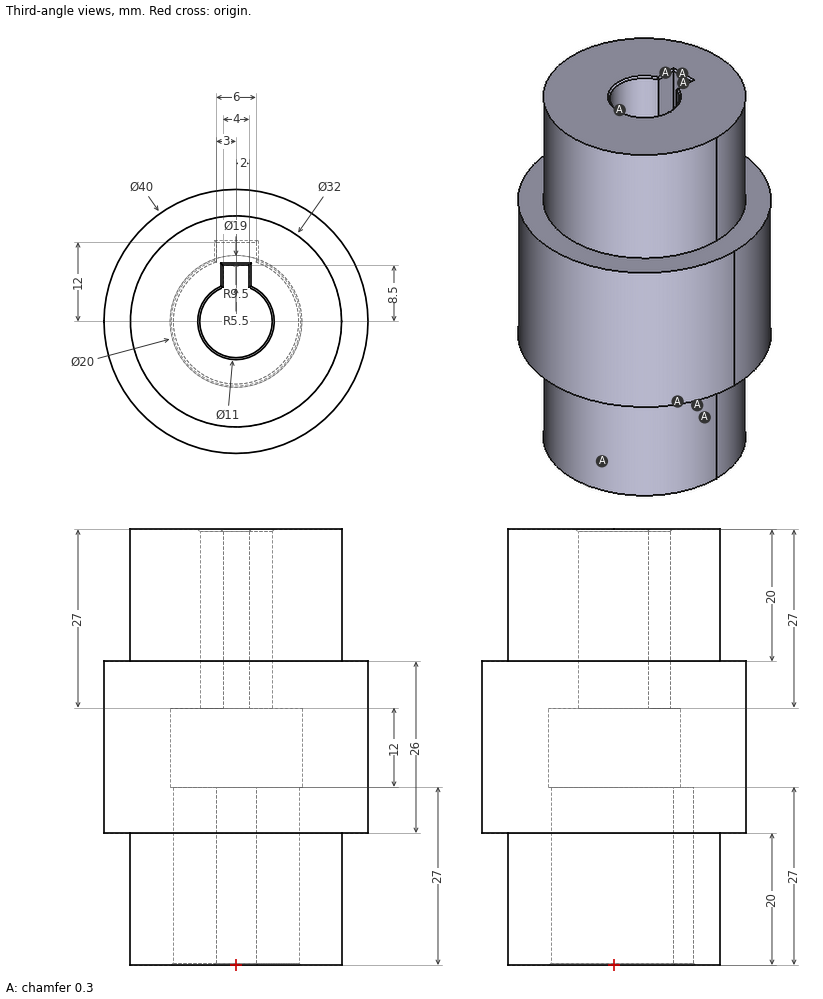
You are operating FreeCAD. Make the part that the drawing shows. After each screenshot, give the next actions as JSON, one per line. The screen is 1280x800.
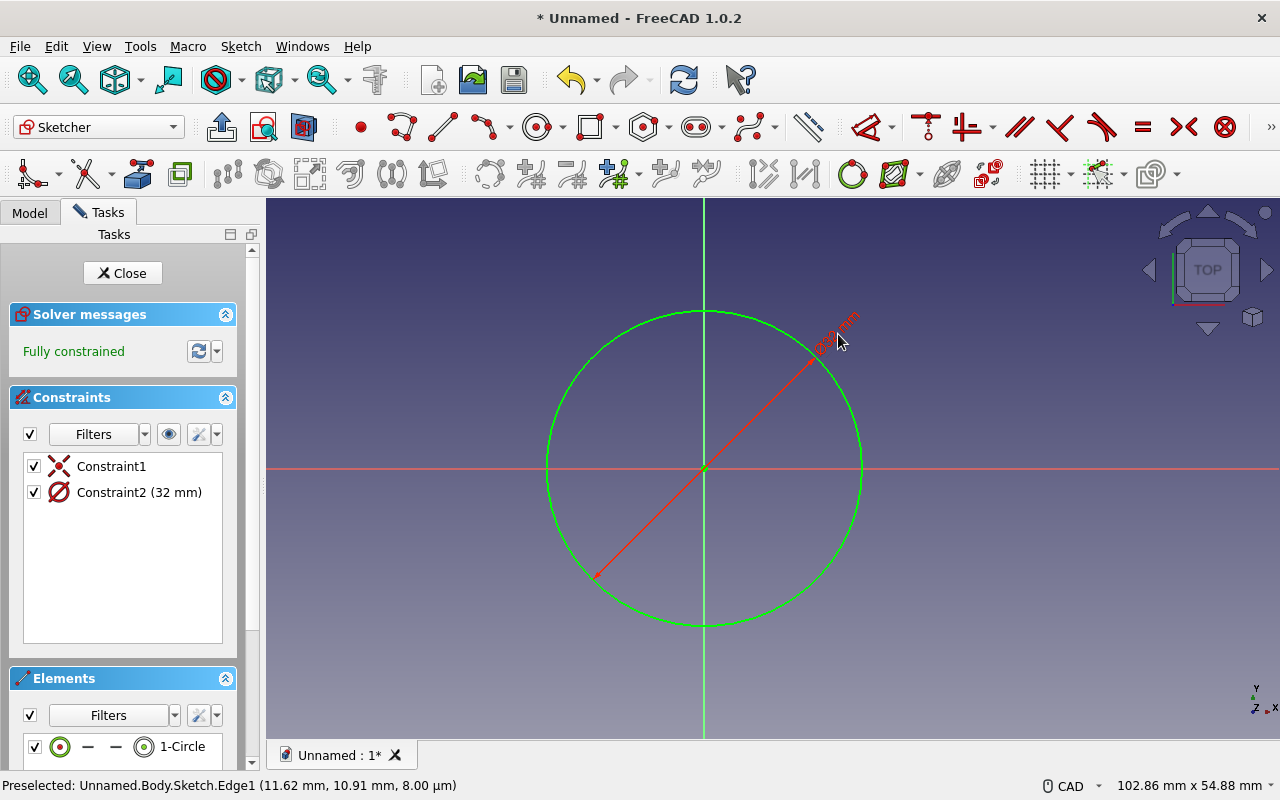
{"action": "left_click", "coordinate": [123, 273]}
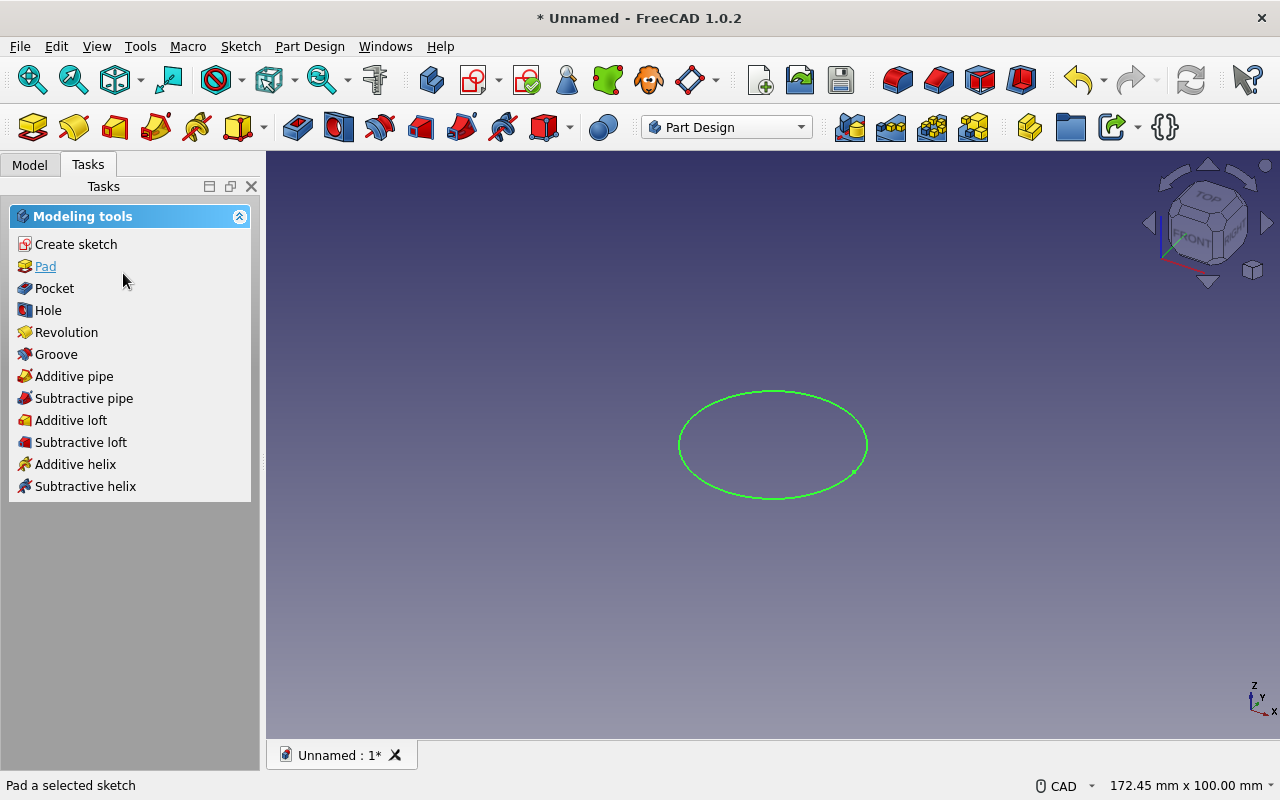
{"action": "left_click", "coordinate": [33, 128]}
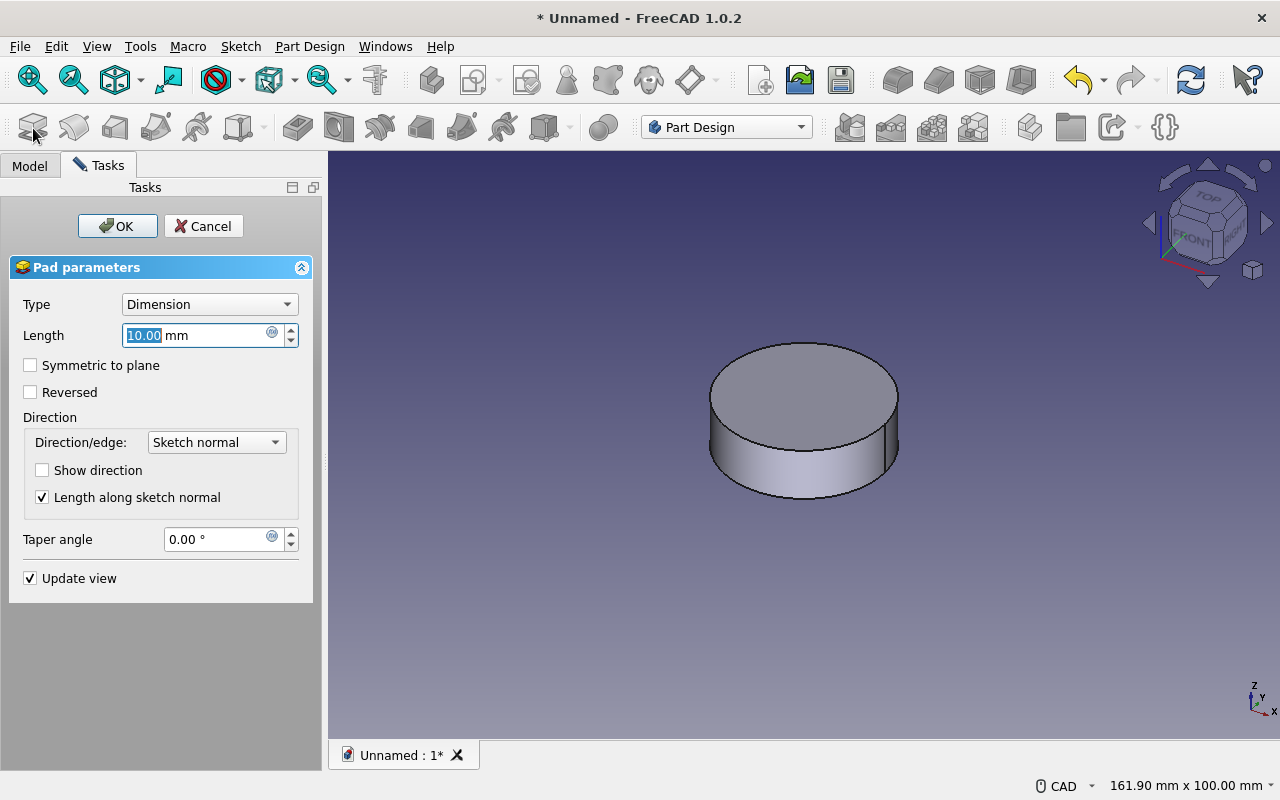
{"action": "type", "text": "20"}
{"action": "key", "text": "Tab"}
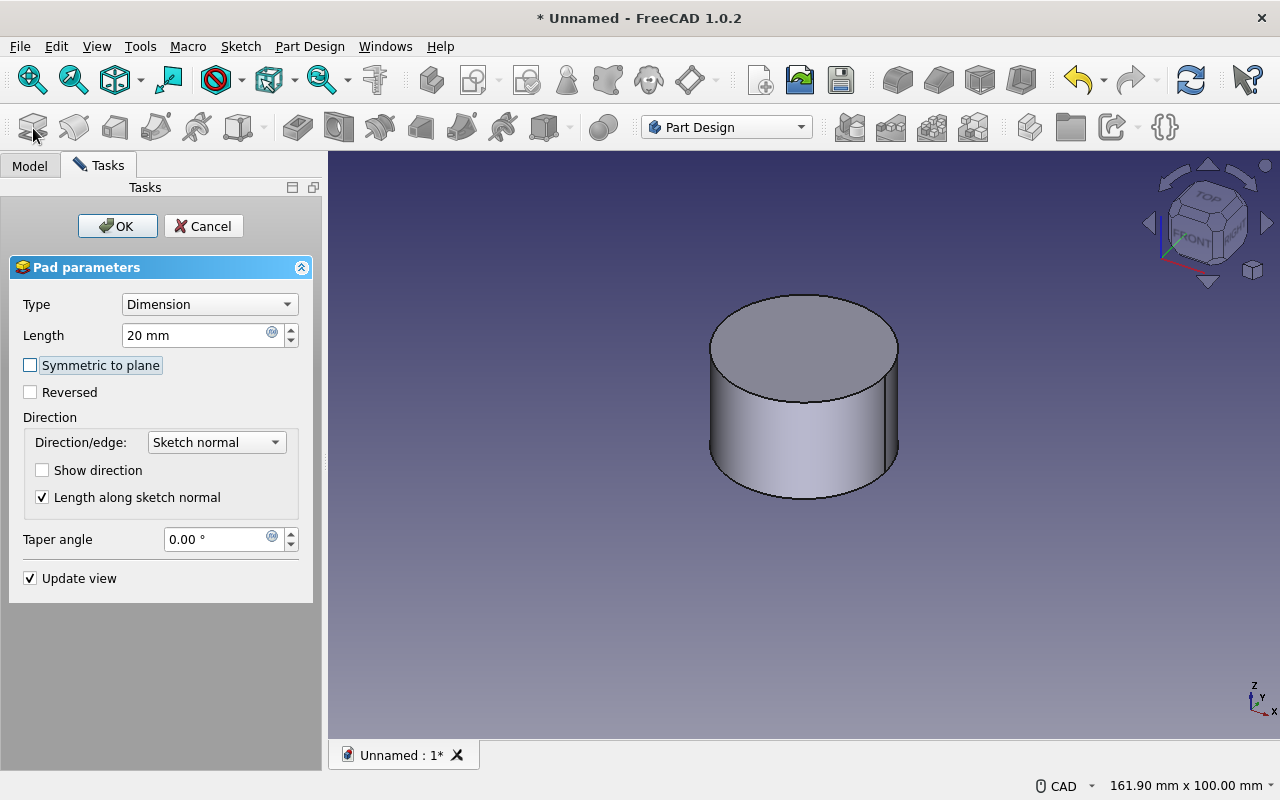
{"action": "left_click", "coordinate": [118, 226]}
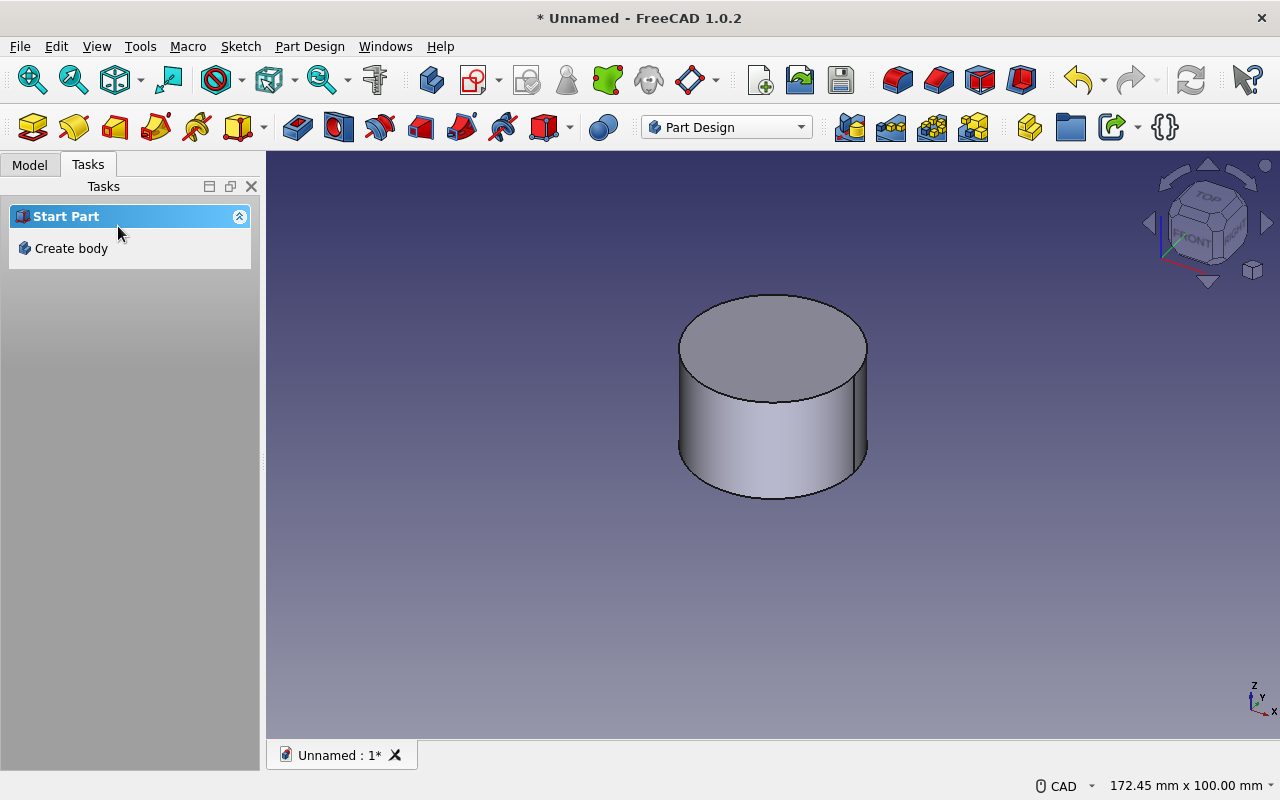
{"action": "left_click", "coordinate": [33, 80]}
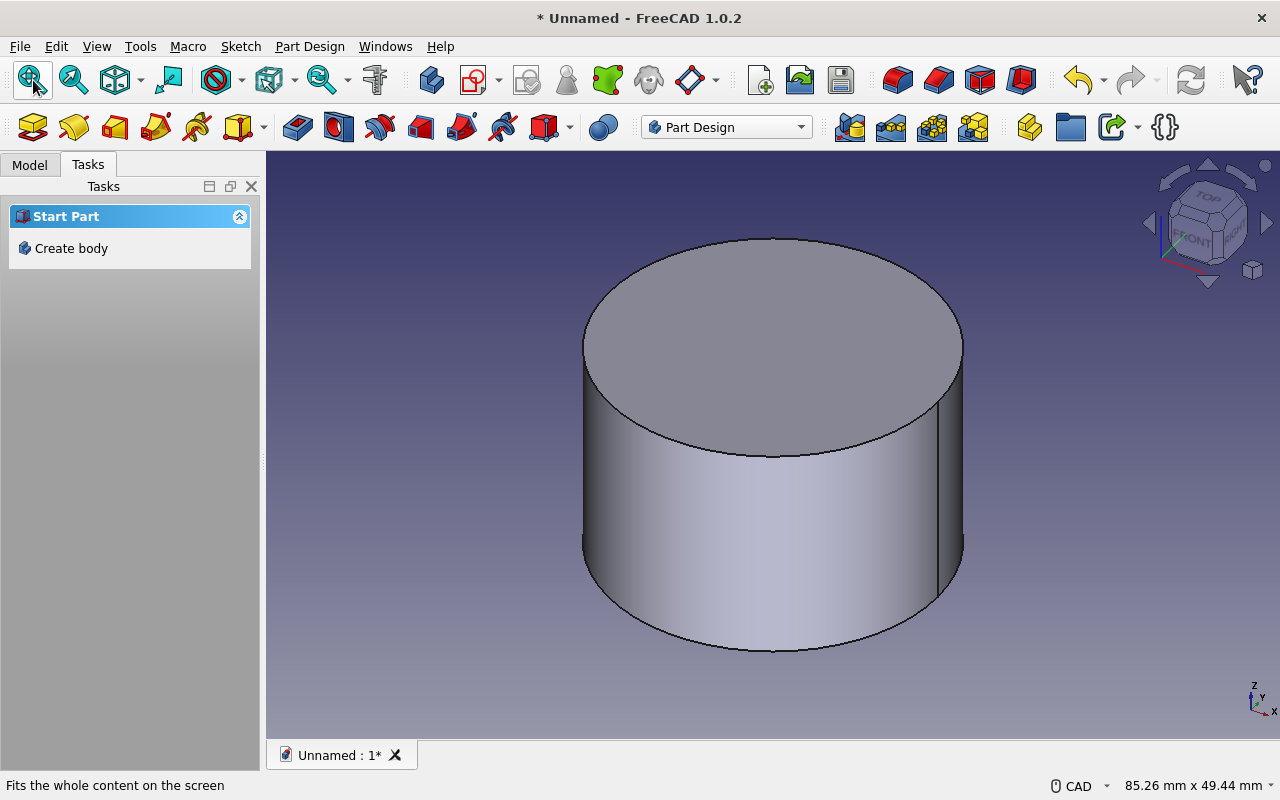
{"action": "left_click", "coordinate": [773, 347]}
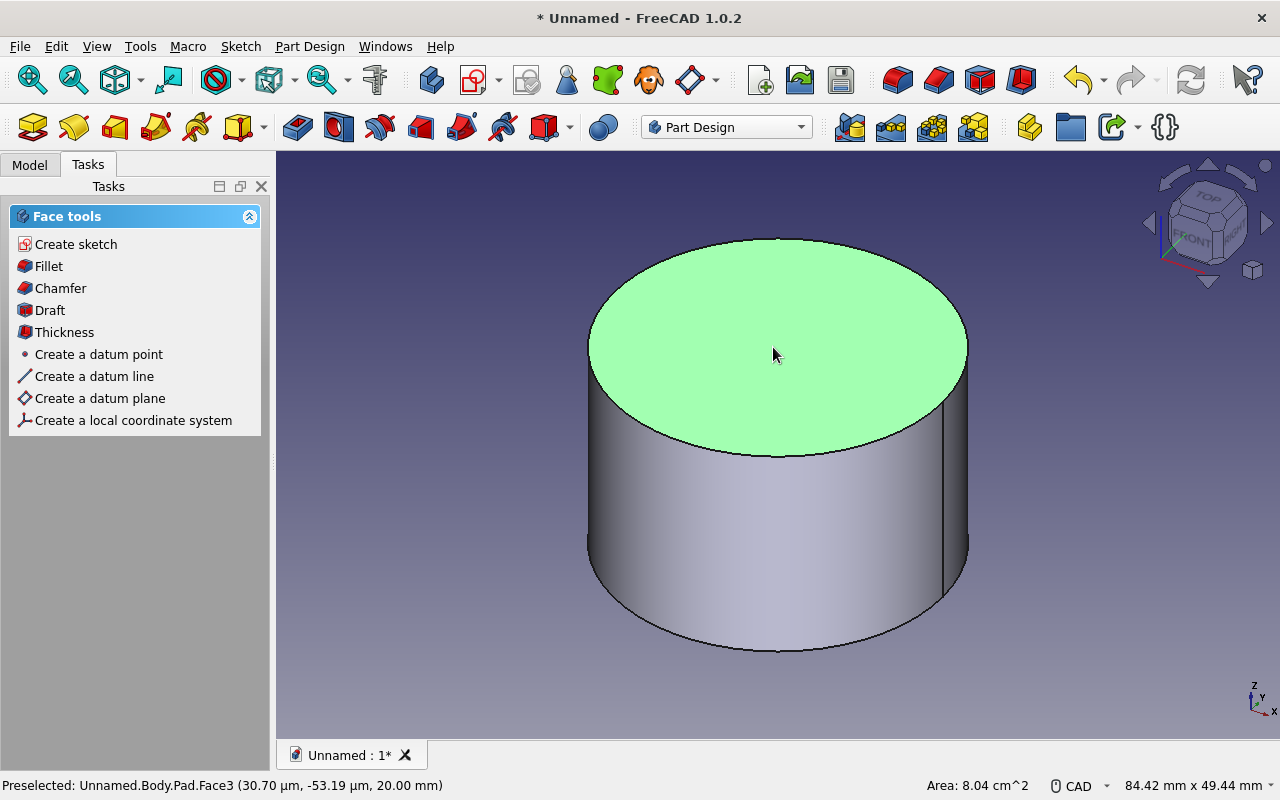
{"action": "left_click", "coordinate": [472, 80]}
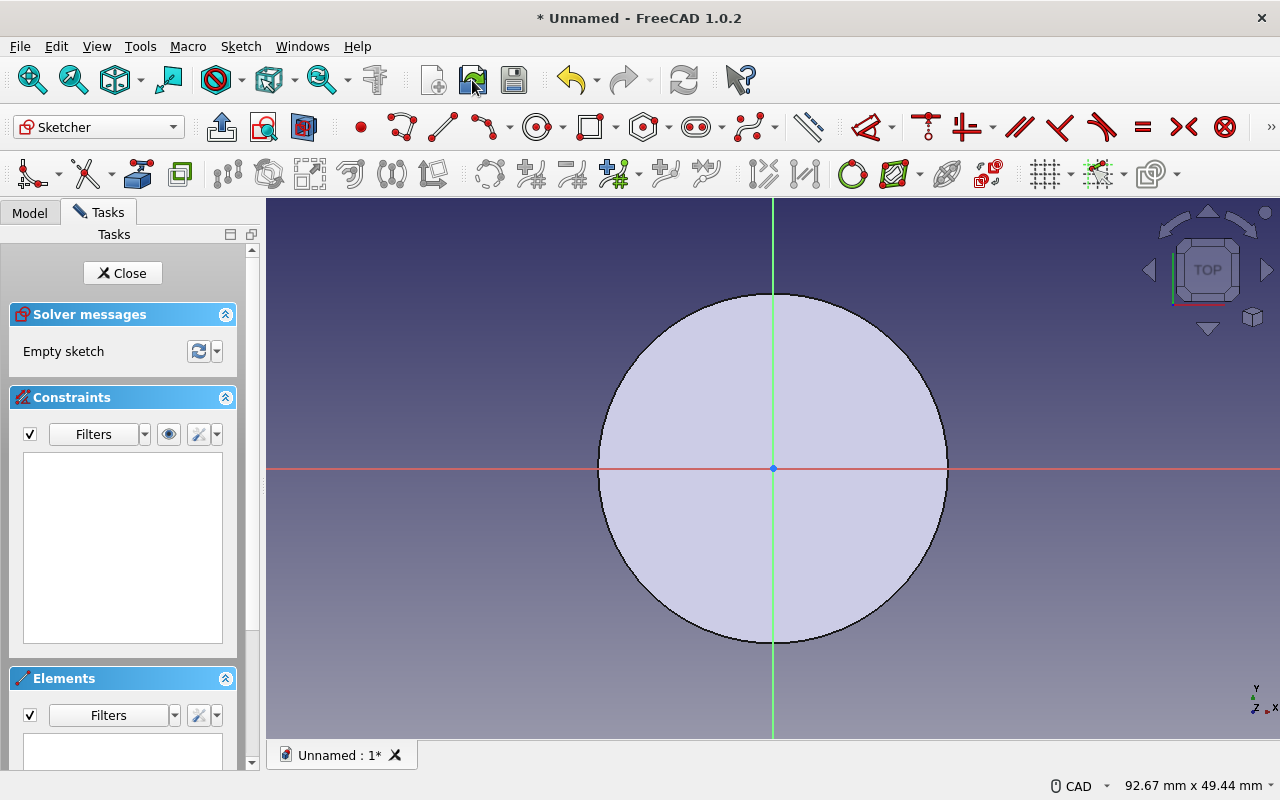
{"action": "scroll", "coordinate": [395, 468], "scroll_direction": "down", "scroll_amount": 1}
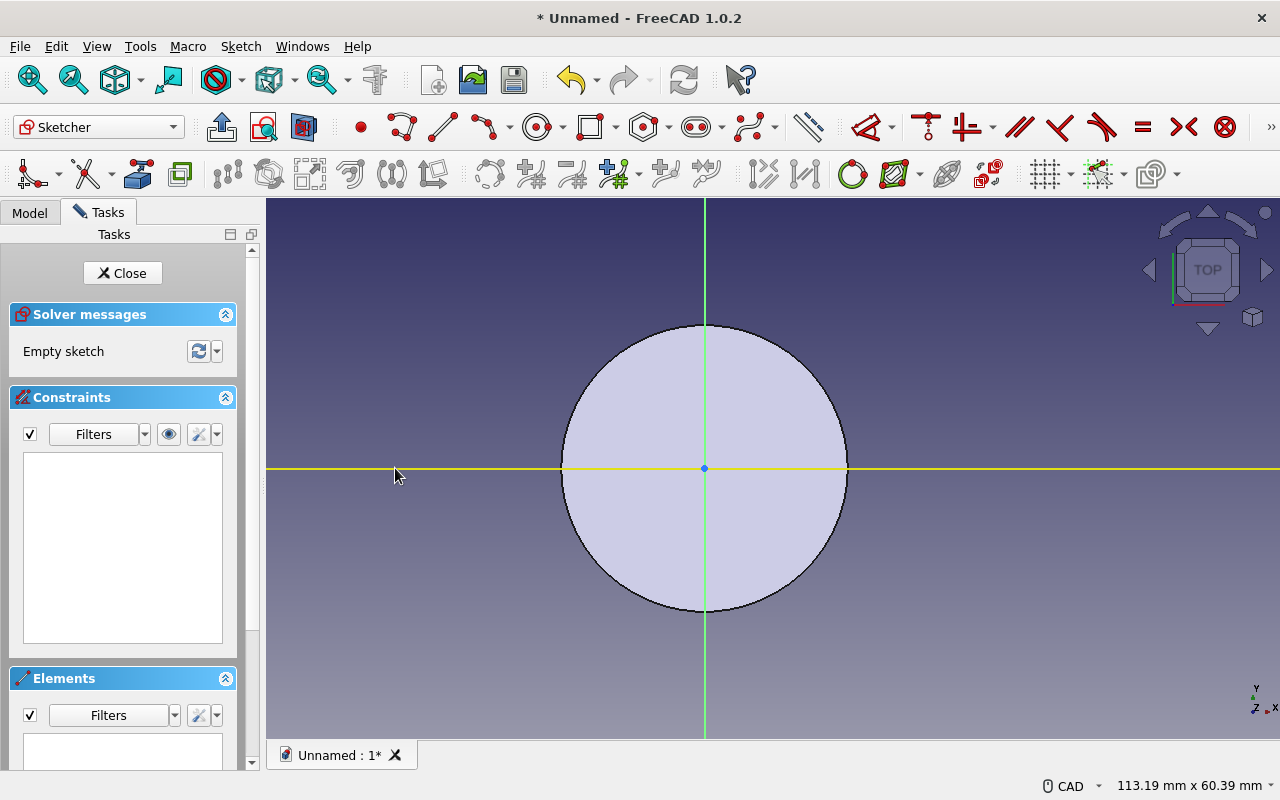
{"action": "left_click", "coordinate": [536, 128]}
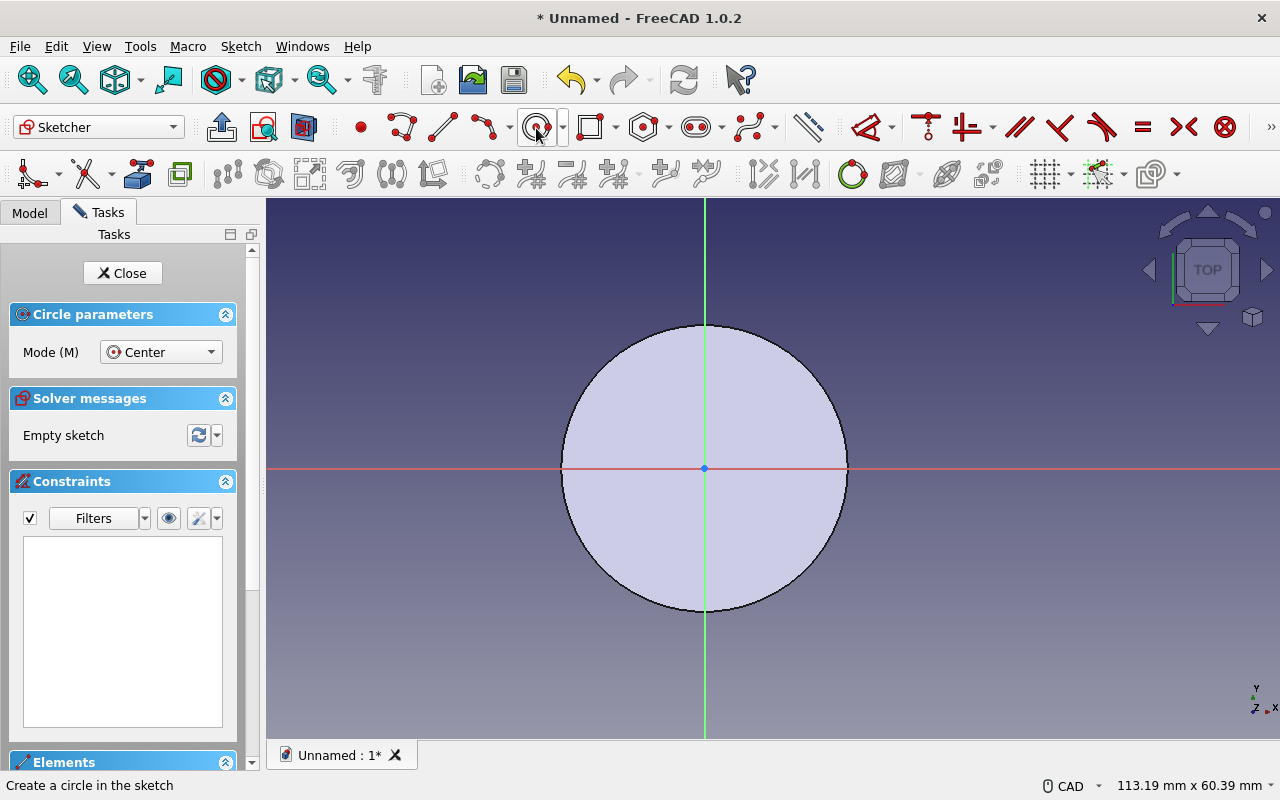
{"action": "left_click", "coordinate": [705, 468]}
{"action": "left_click", "coordinate": [831, 342]}
{"action": "key", "text": "Escape"}